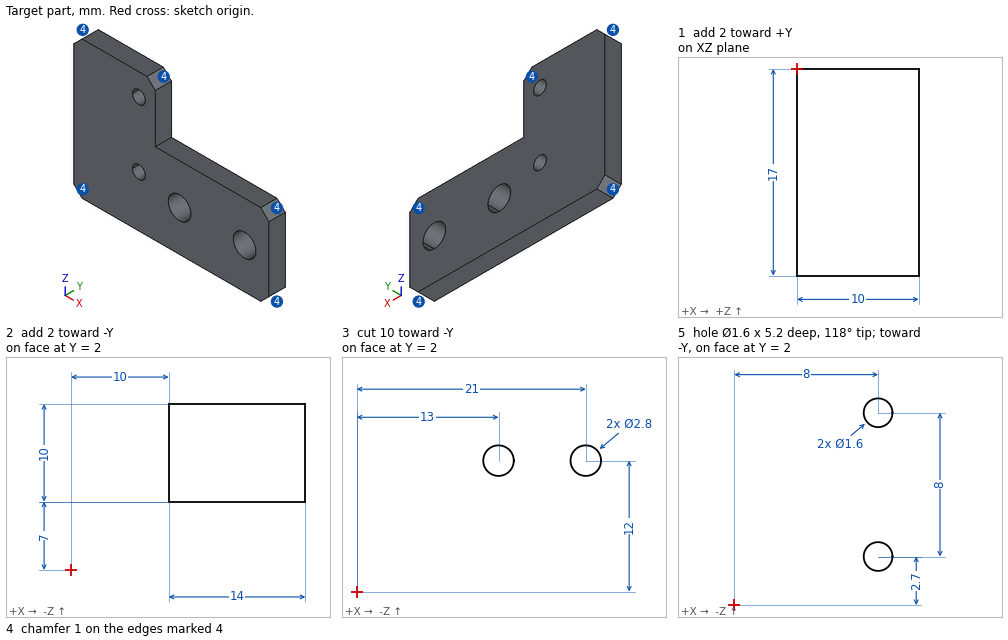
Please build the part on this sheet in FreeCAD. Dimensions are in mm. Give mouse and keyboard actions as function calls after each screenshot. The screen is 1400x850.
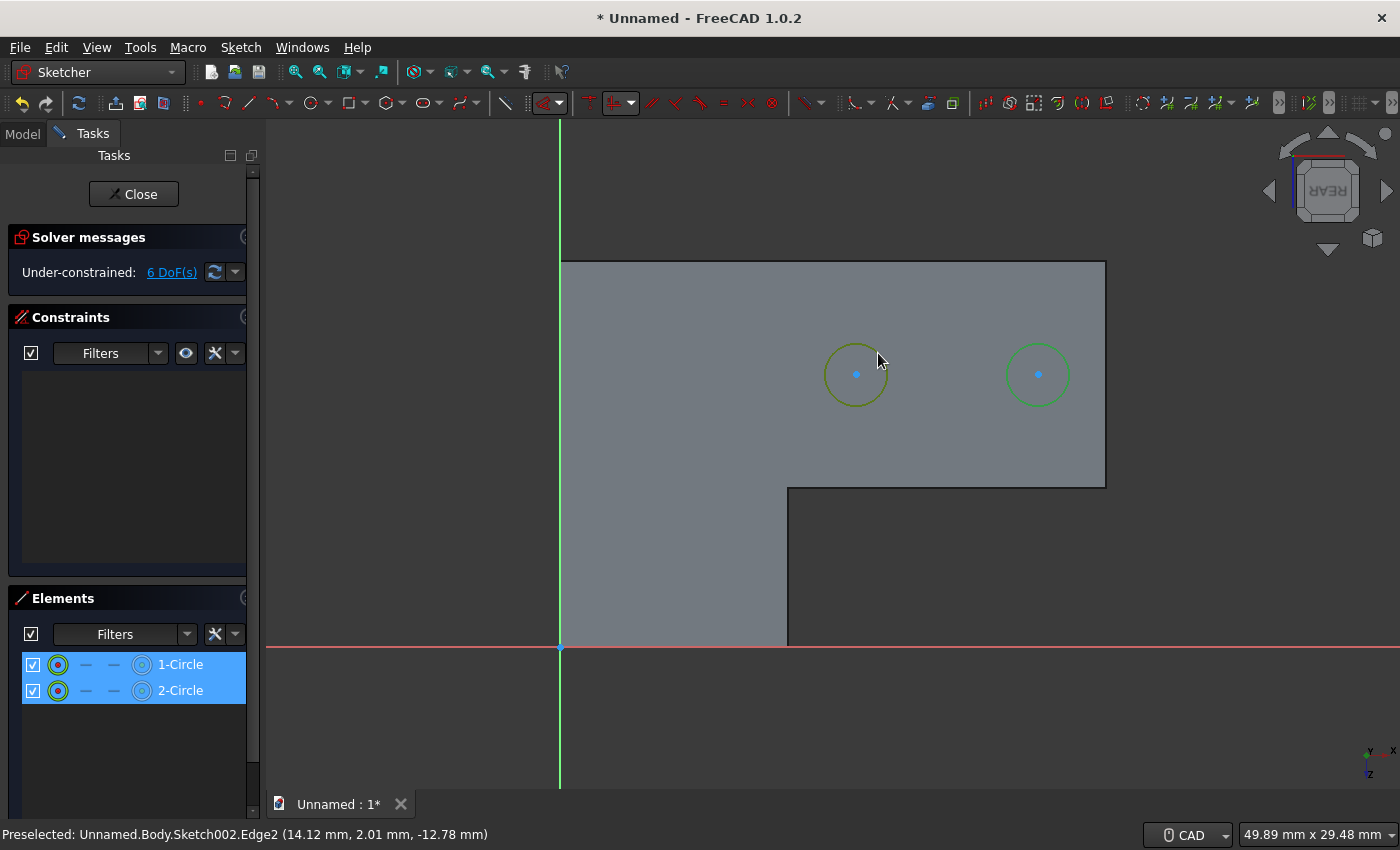
click(724, 104)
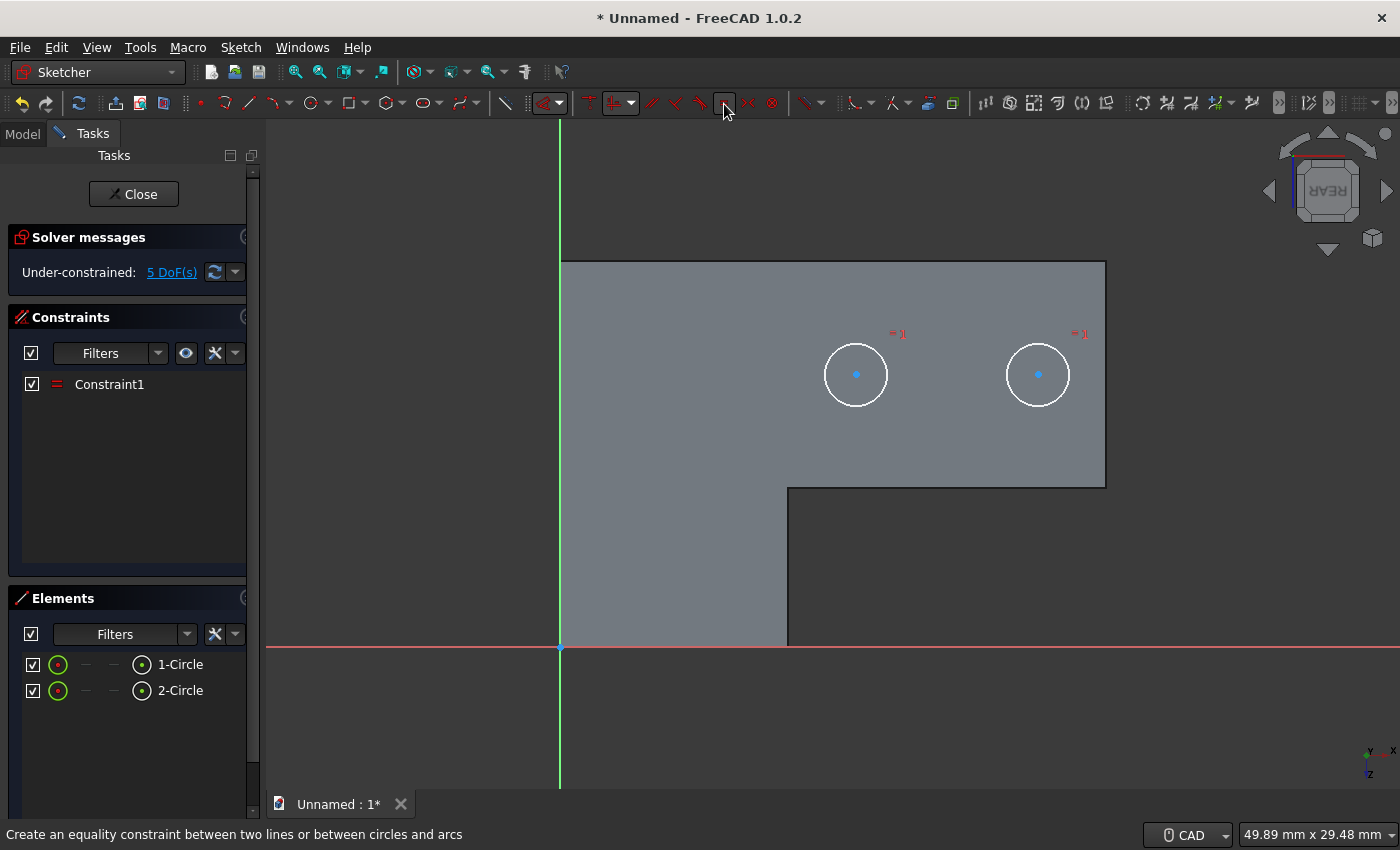
click(1038, 375)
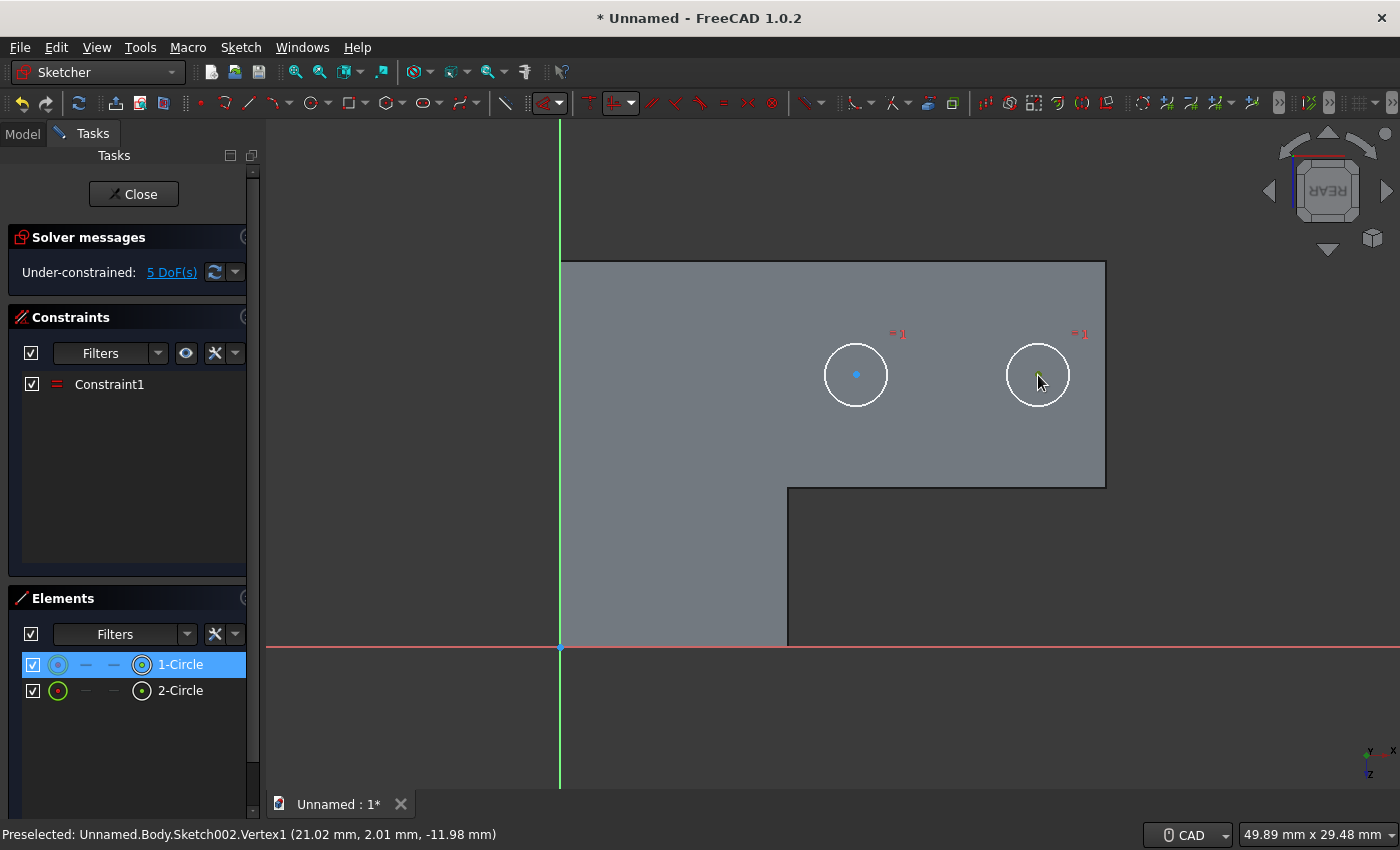
click(856, 375)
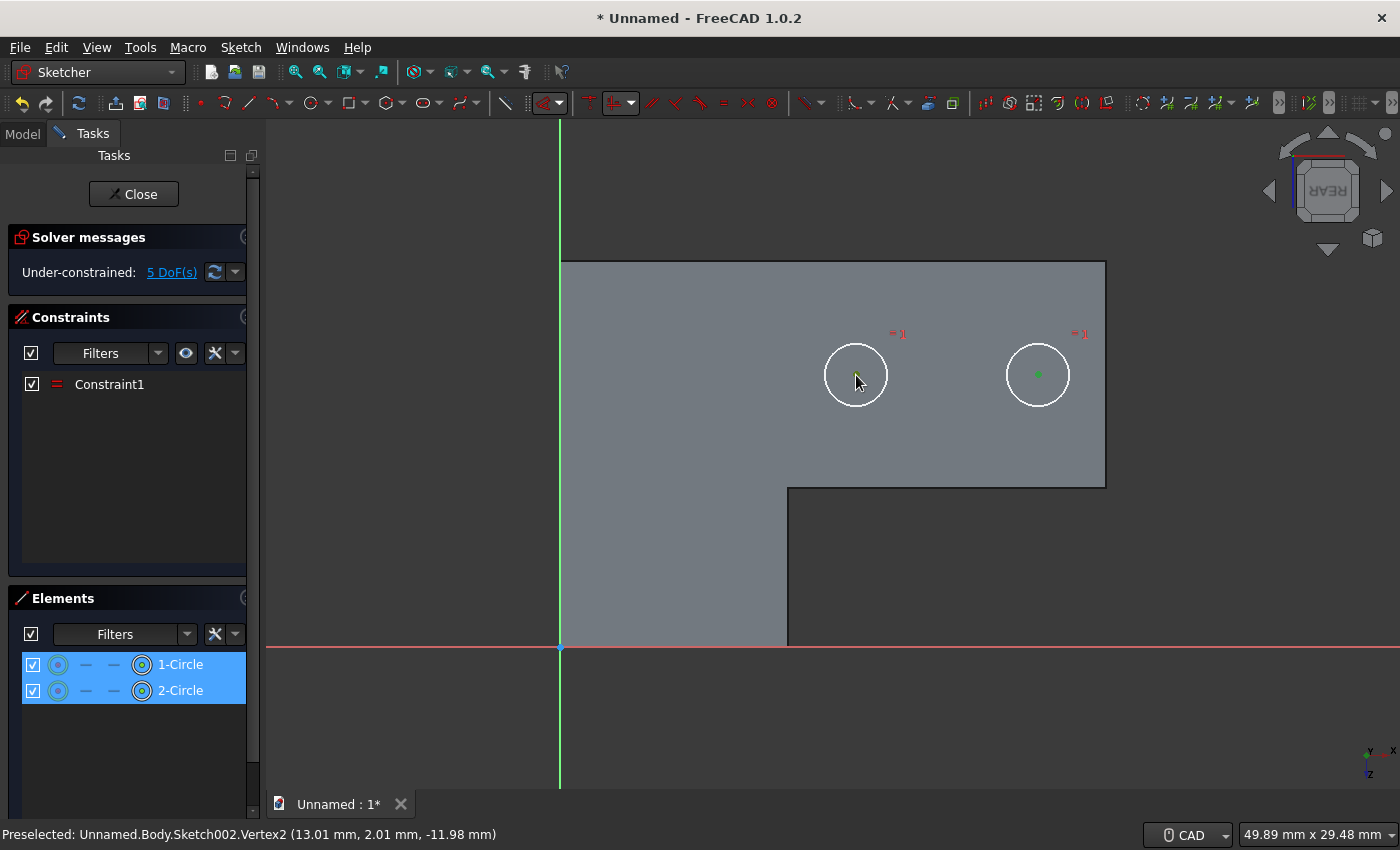
key(h)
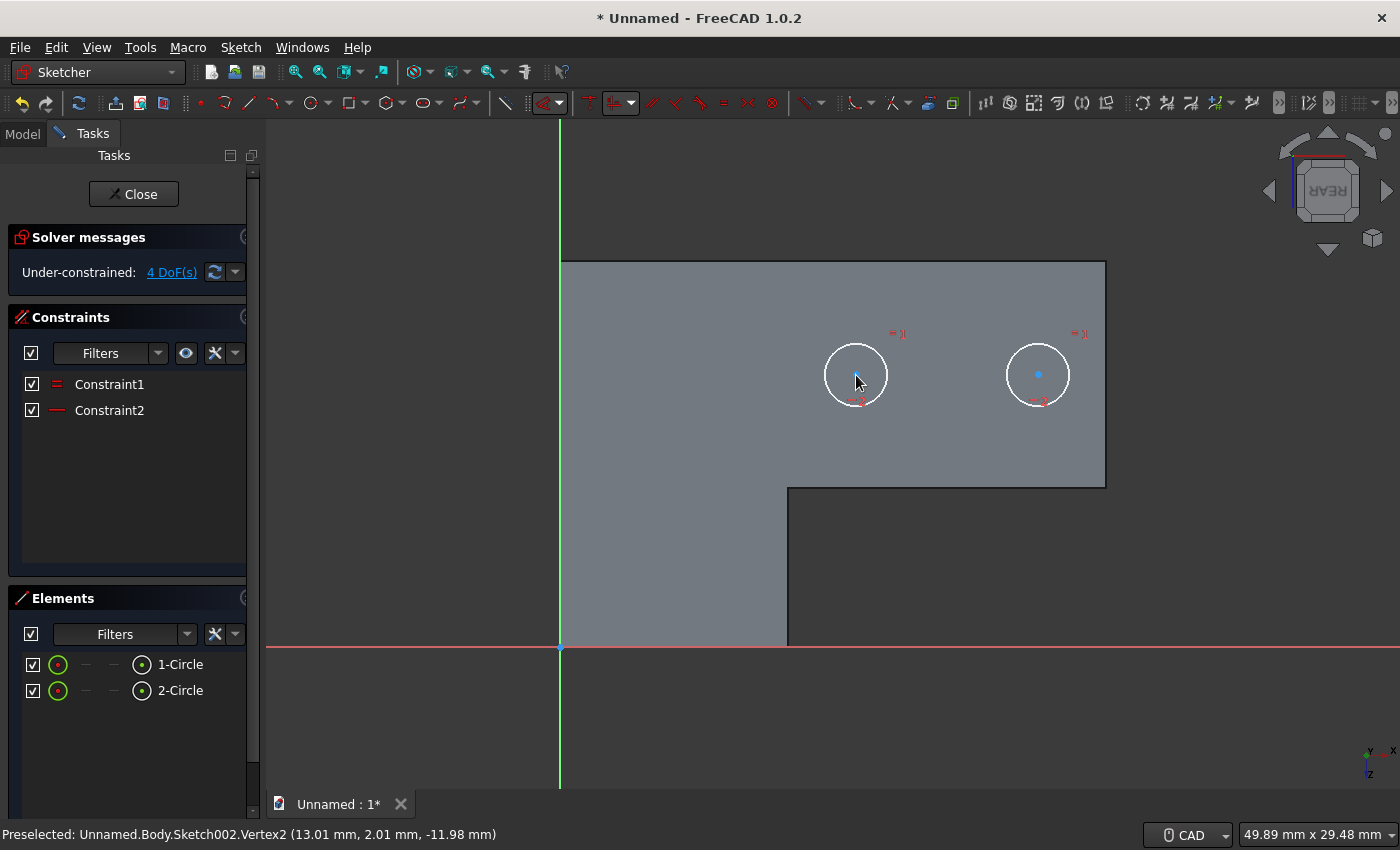
click(1060, 353)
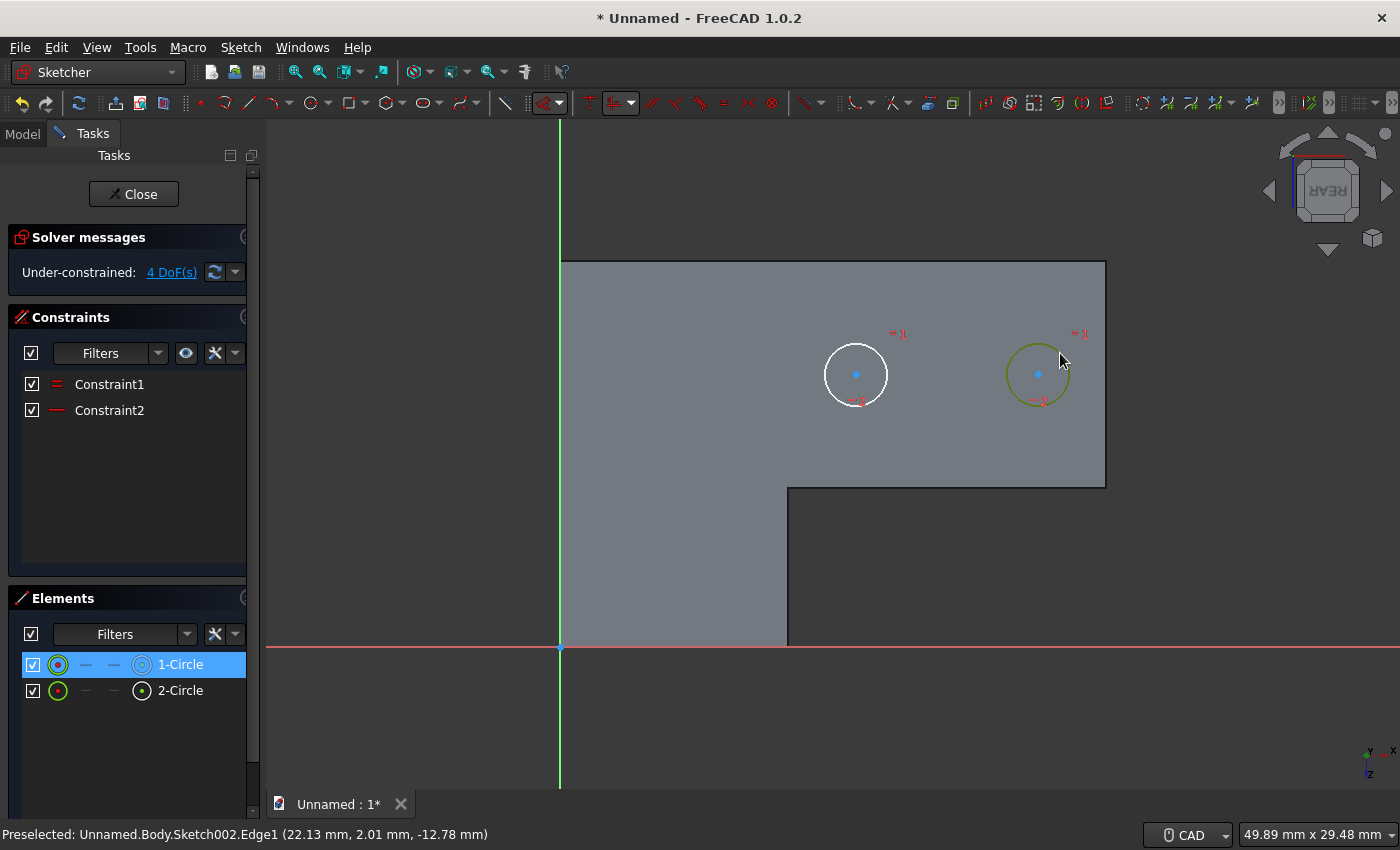
click(562, 104)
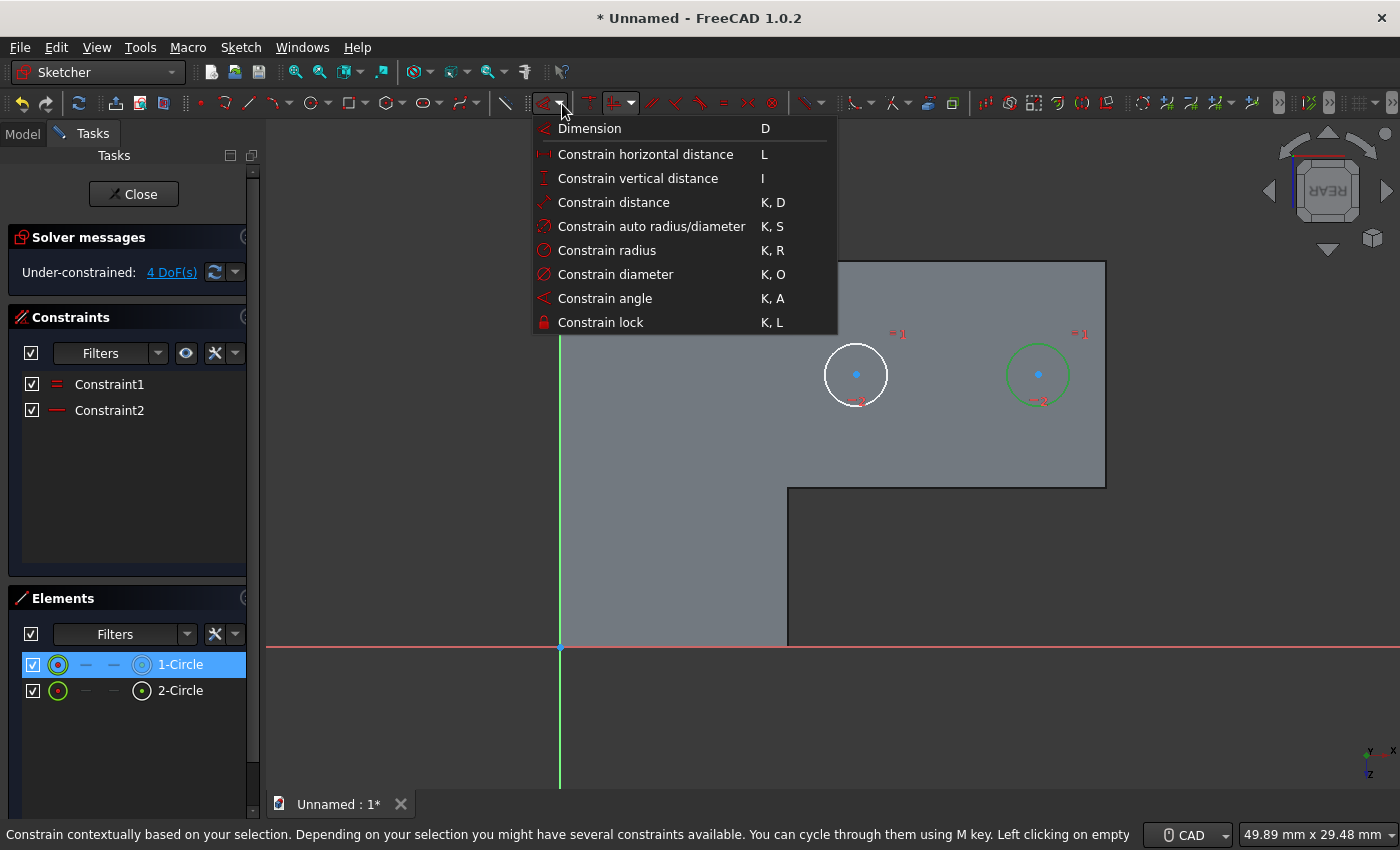
click(685, 274)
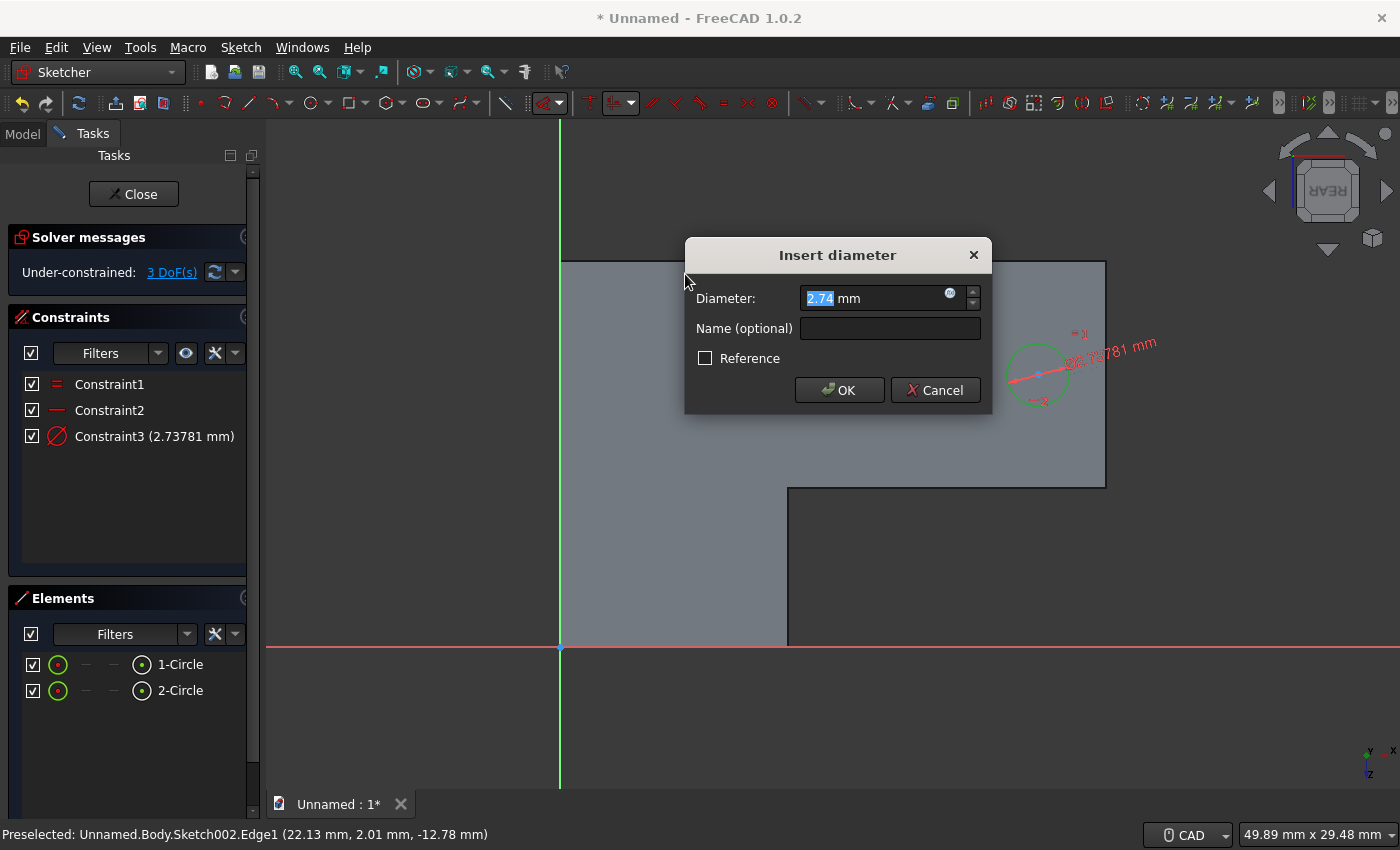
text(2.8)
key(Return)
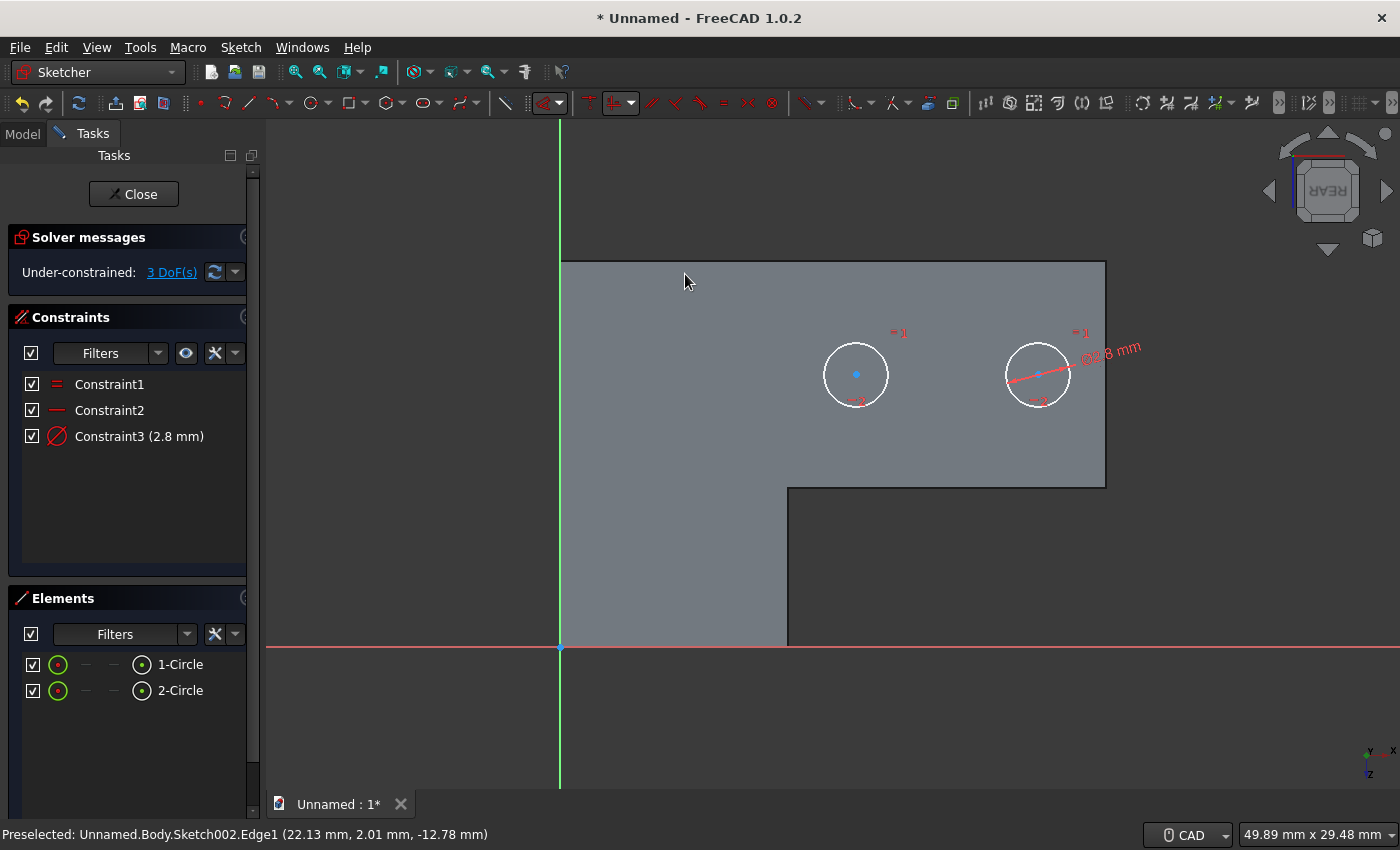
click(1038, 375)